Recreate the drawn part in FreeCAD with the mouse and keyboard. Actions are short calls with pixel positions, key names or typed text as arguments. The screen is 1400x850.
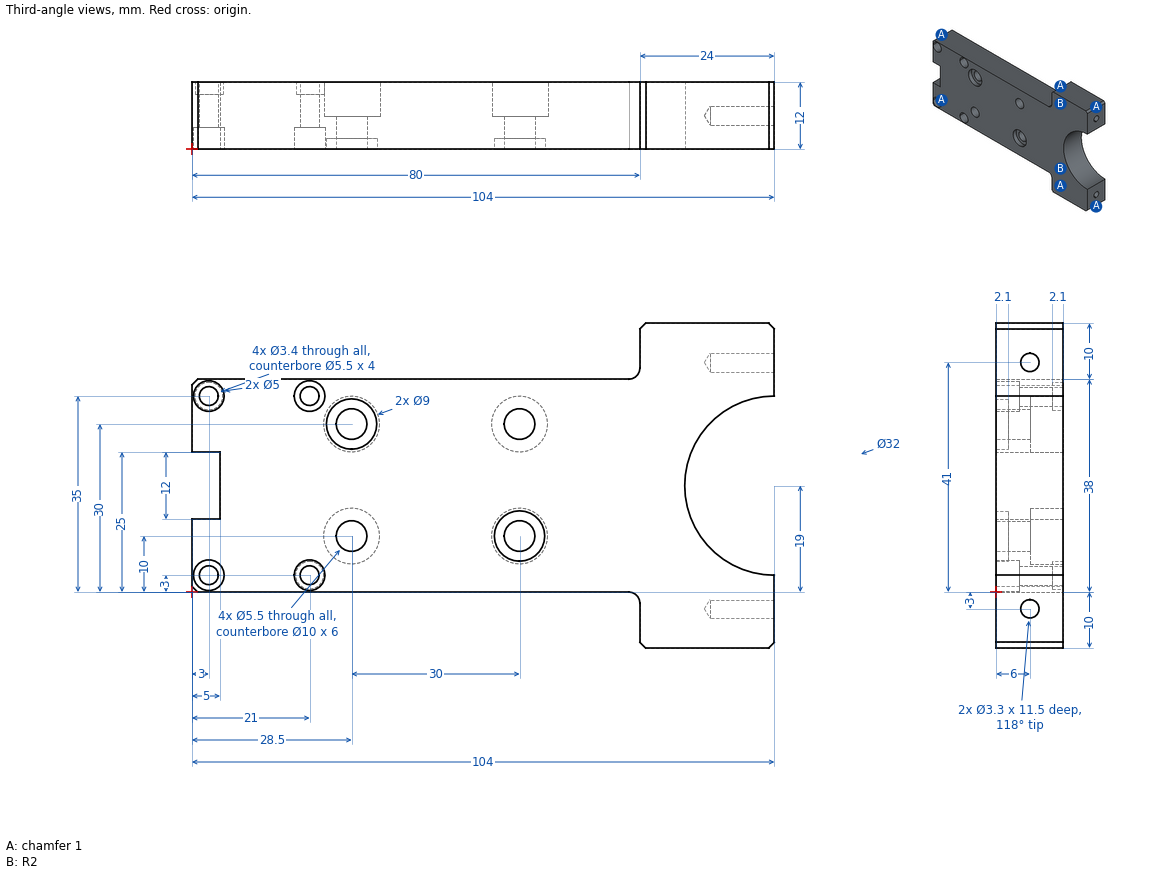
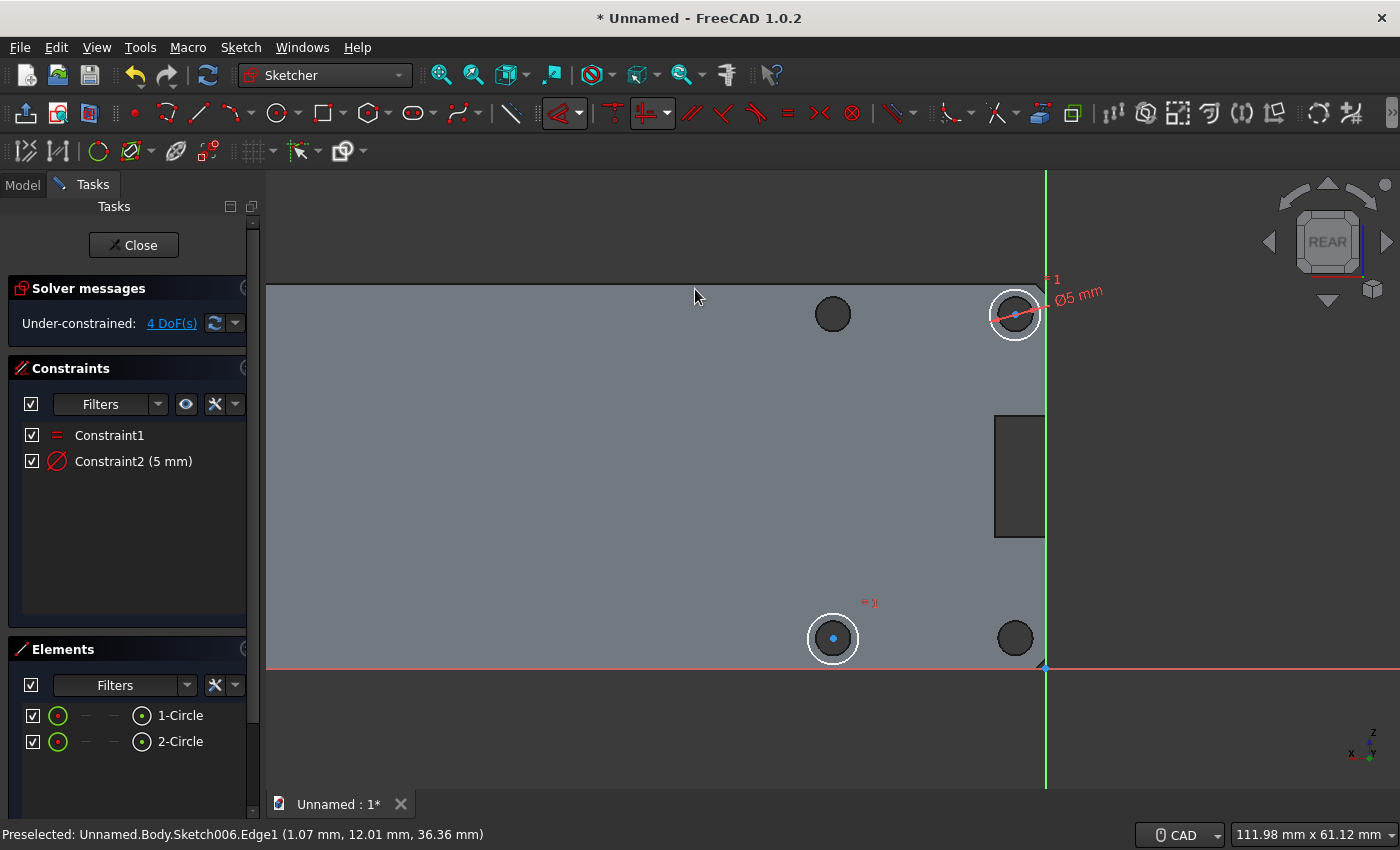
scroll(1015, 315, up, 2)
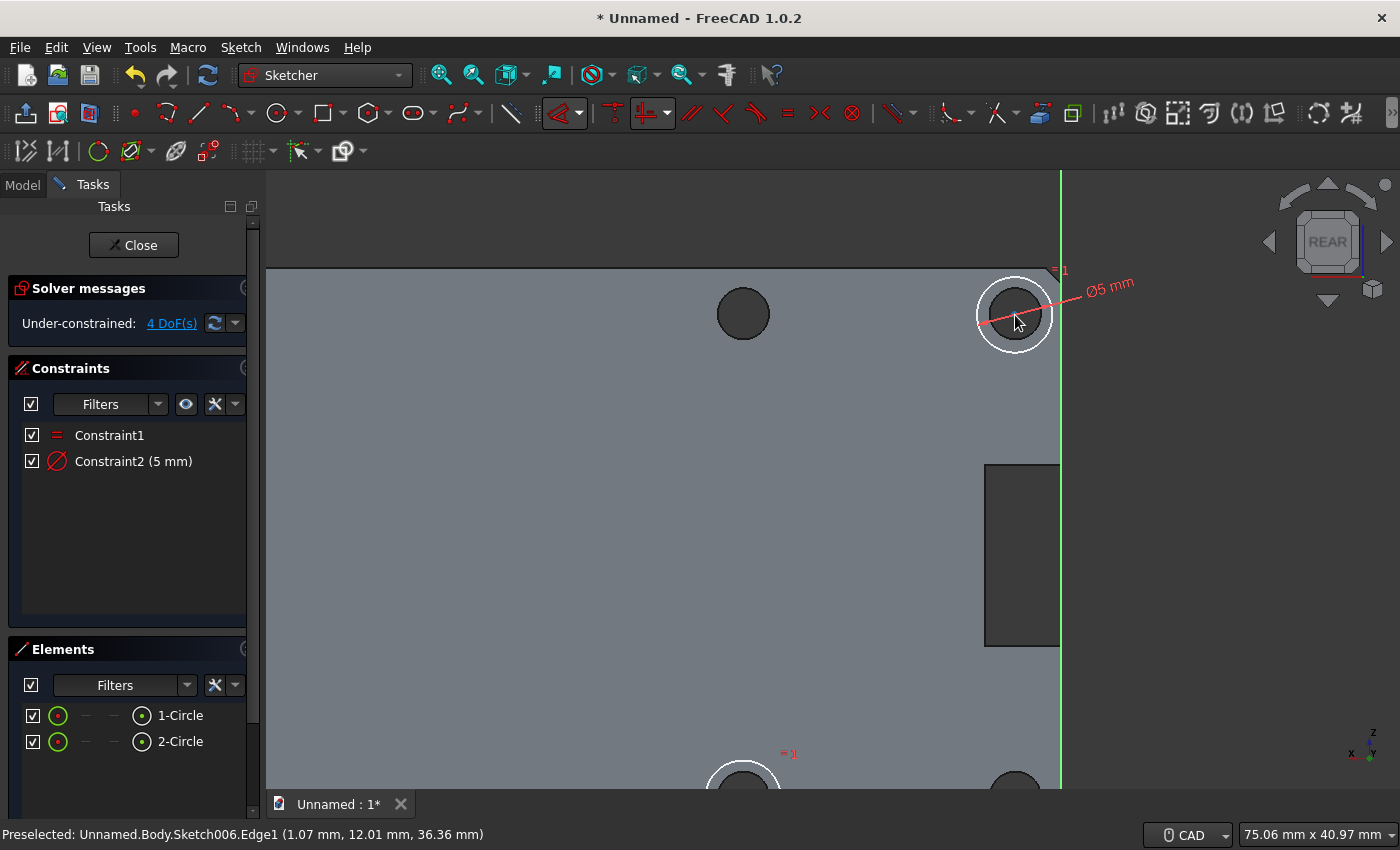
click(1015, 315)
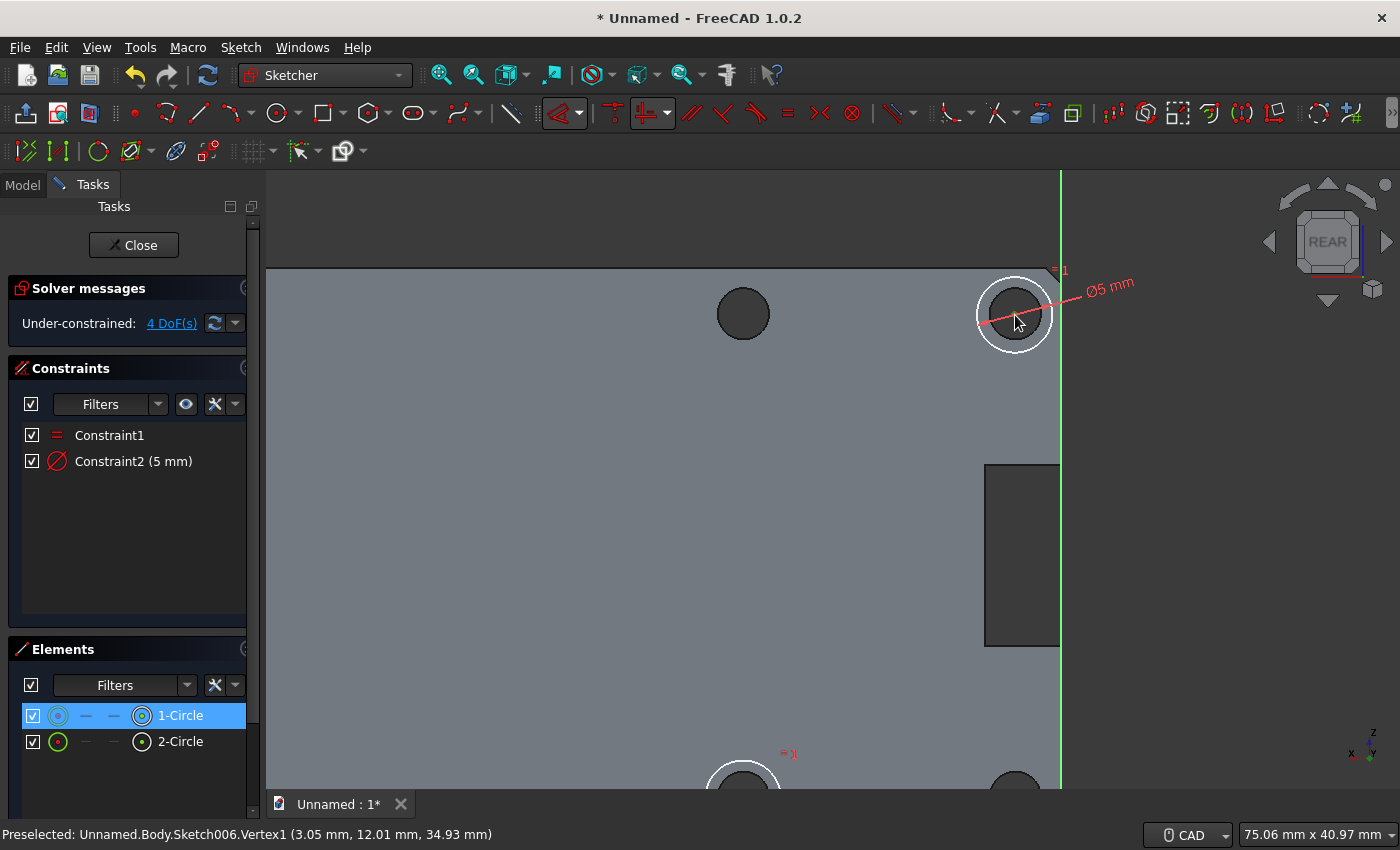
key(l)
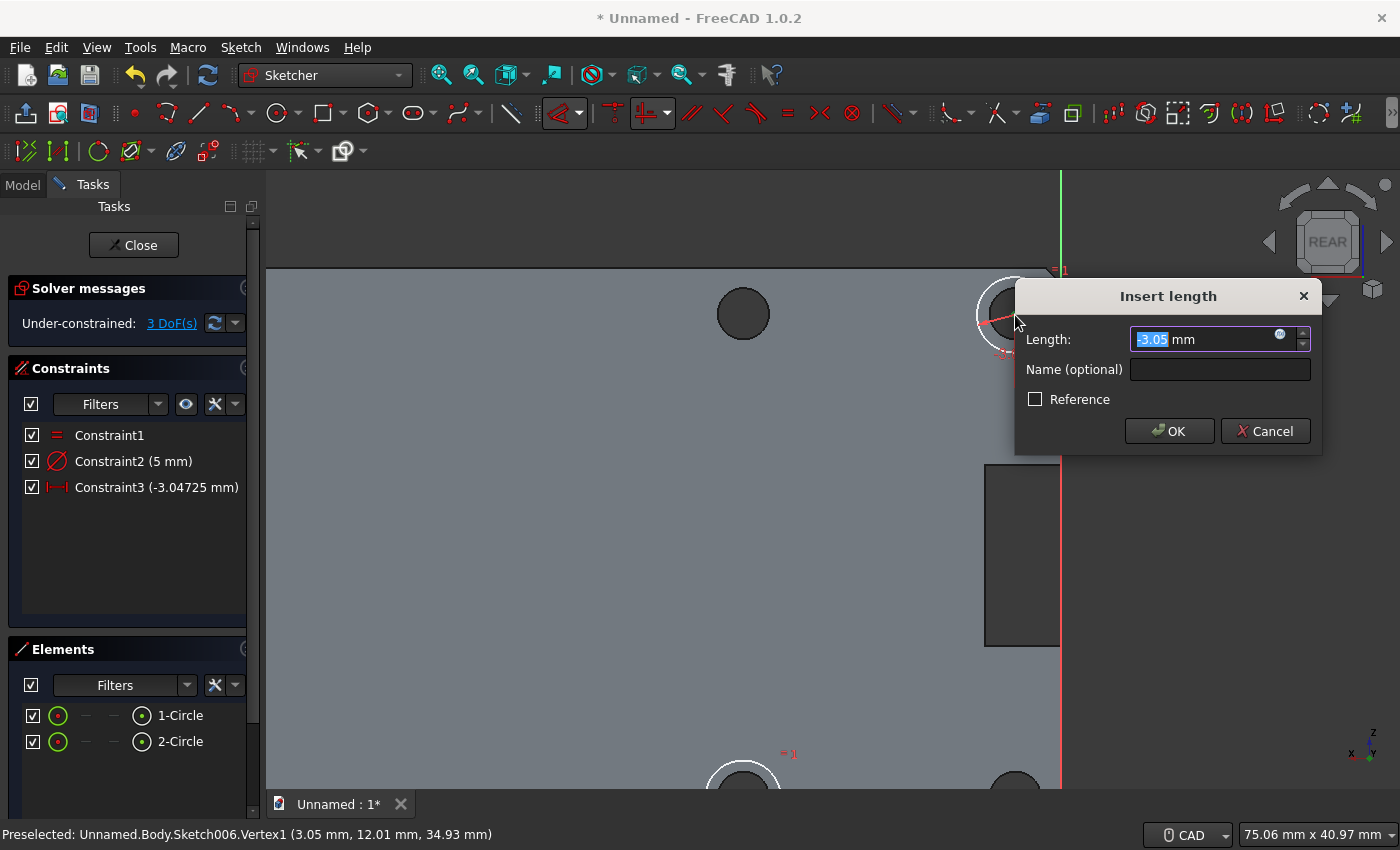
text(-3)
key(Return)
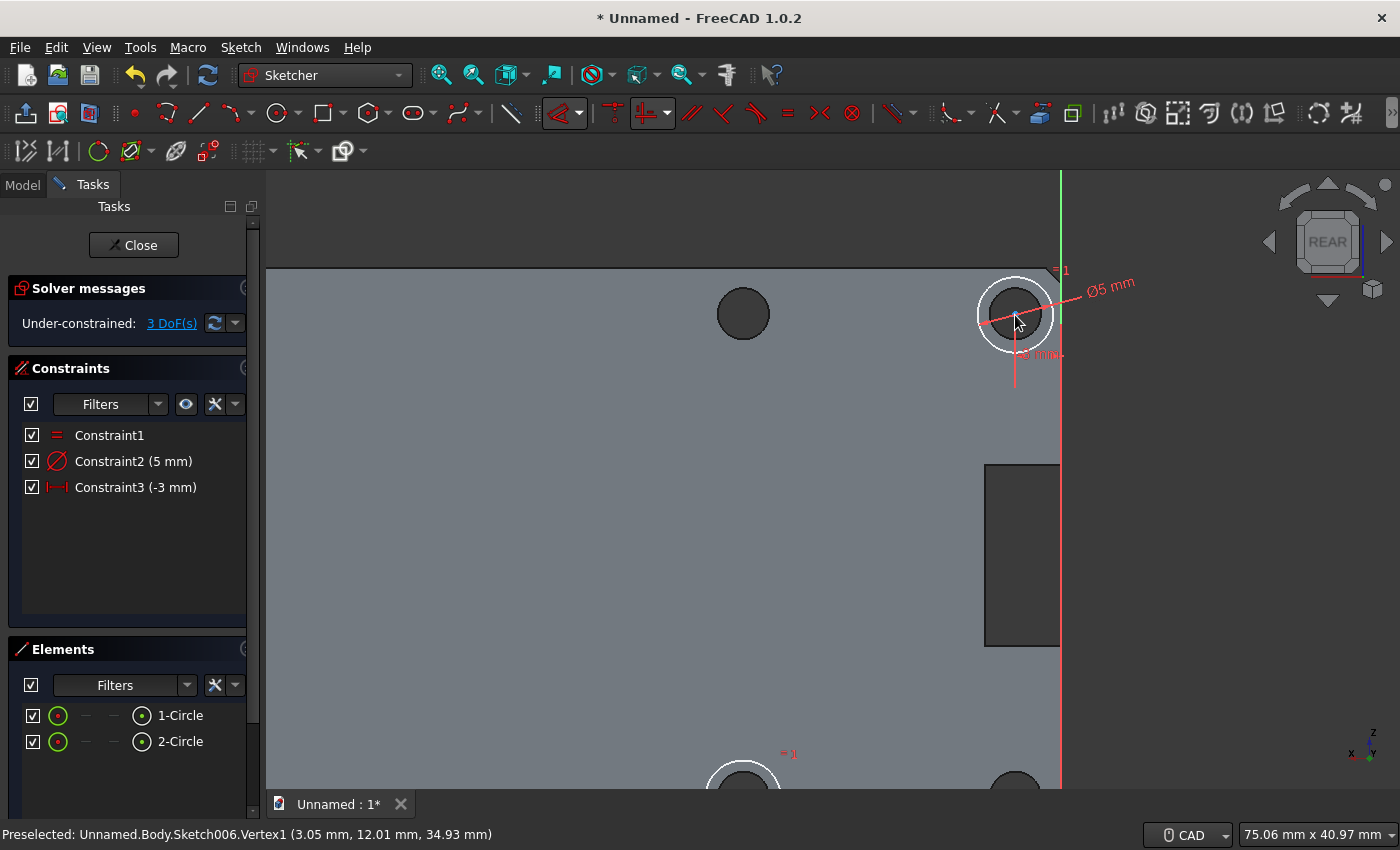
scroll(523, 317, down, 2)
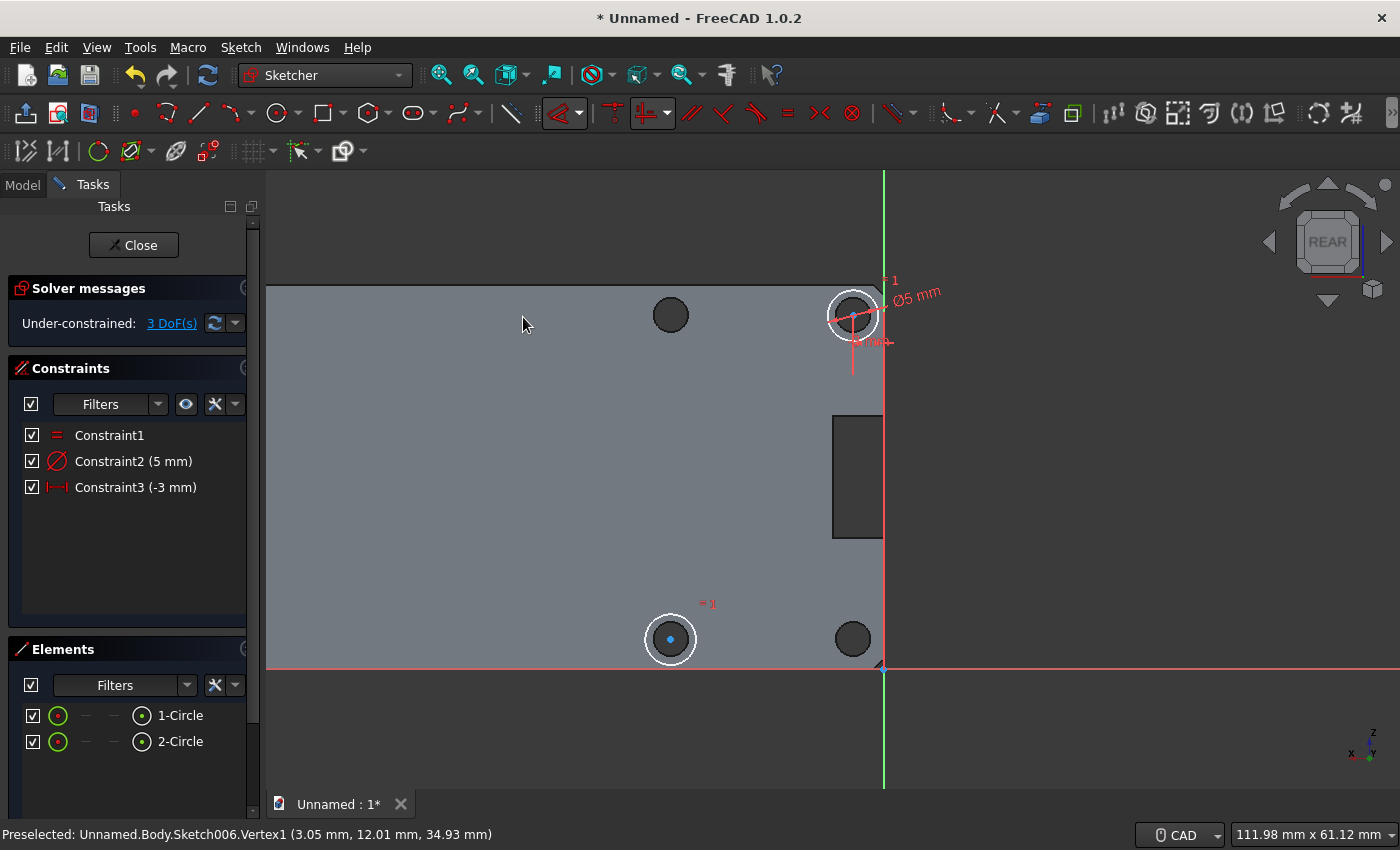
scroll(671, 640, up, 2)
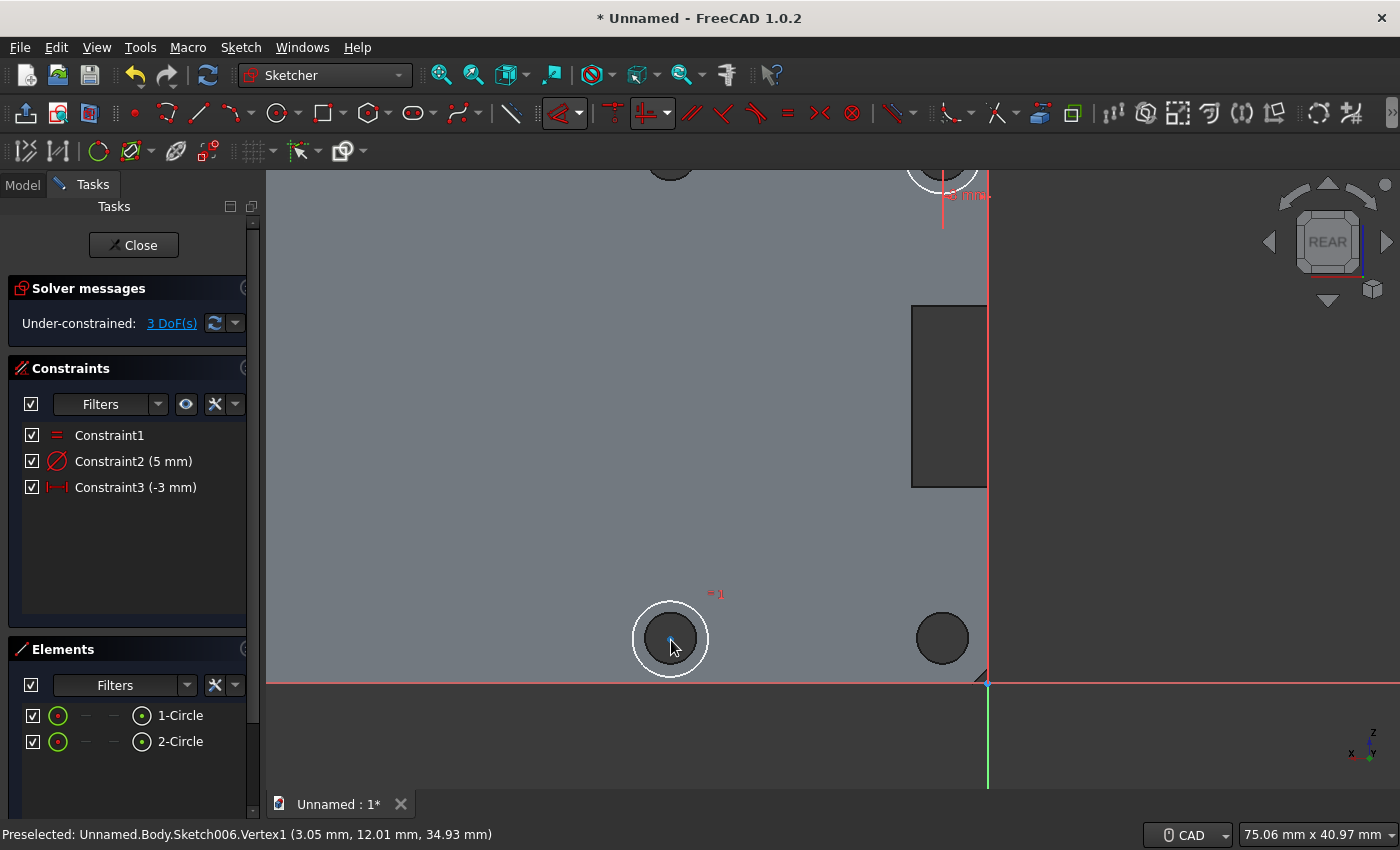
click(670, 639)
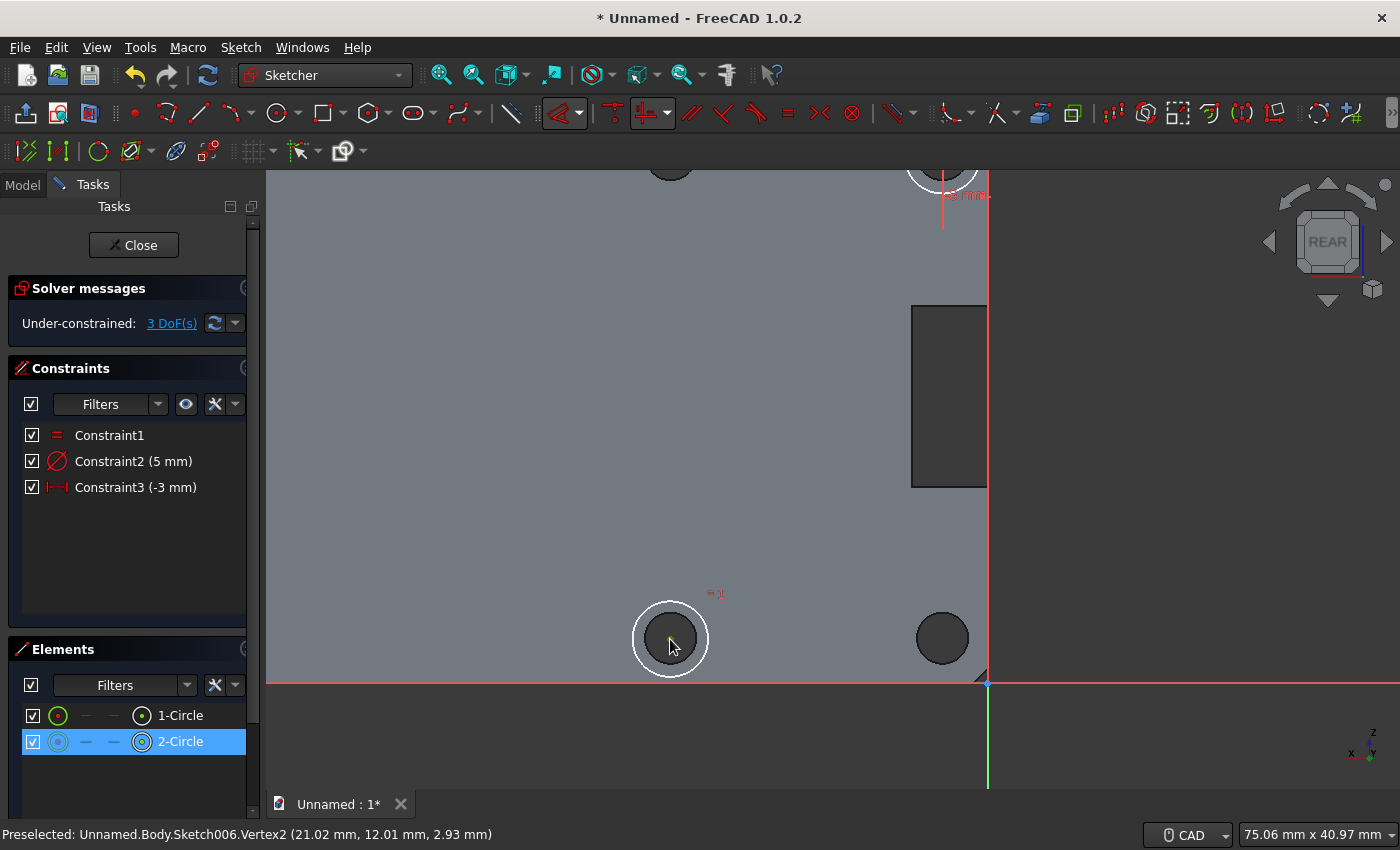
key(i)